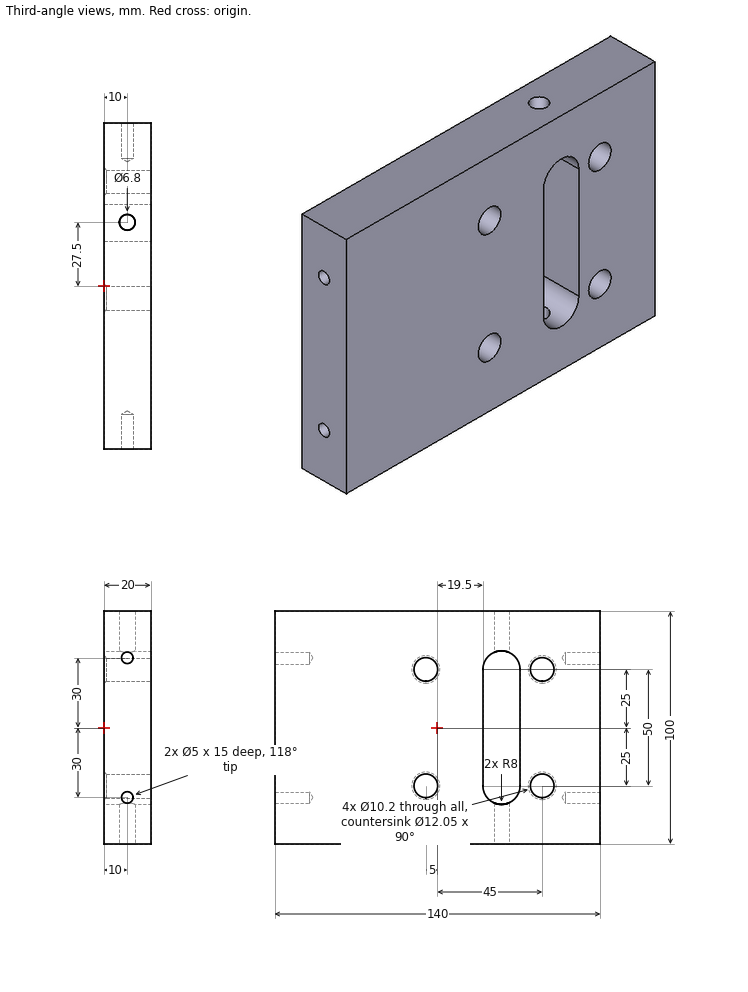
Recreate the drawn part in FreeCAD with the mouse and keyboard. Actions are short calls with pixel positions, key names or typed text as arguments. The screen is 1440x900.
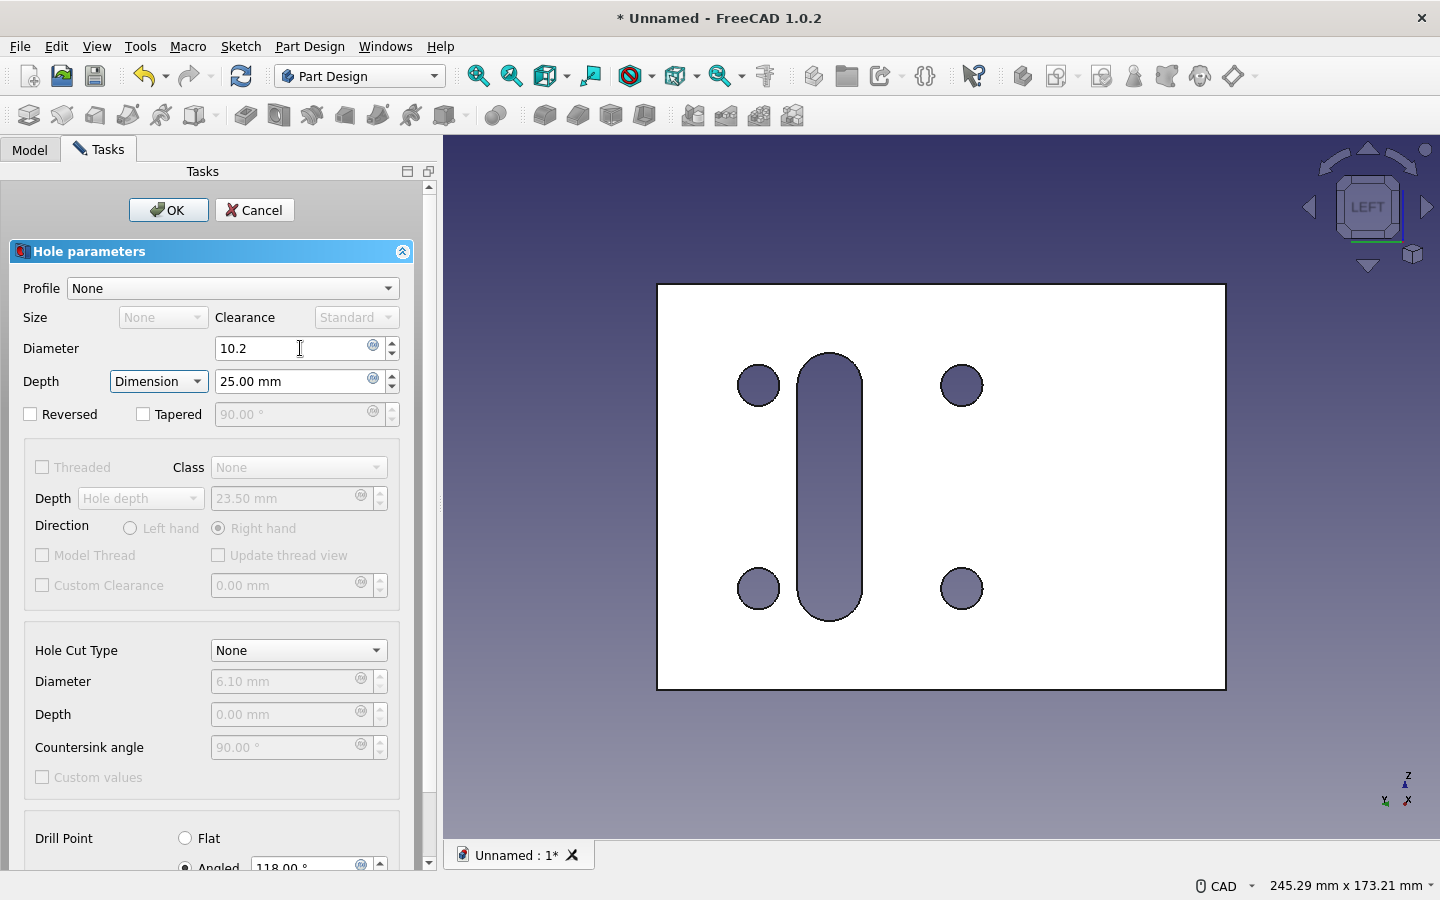
click(160, 382)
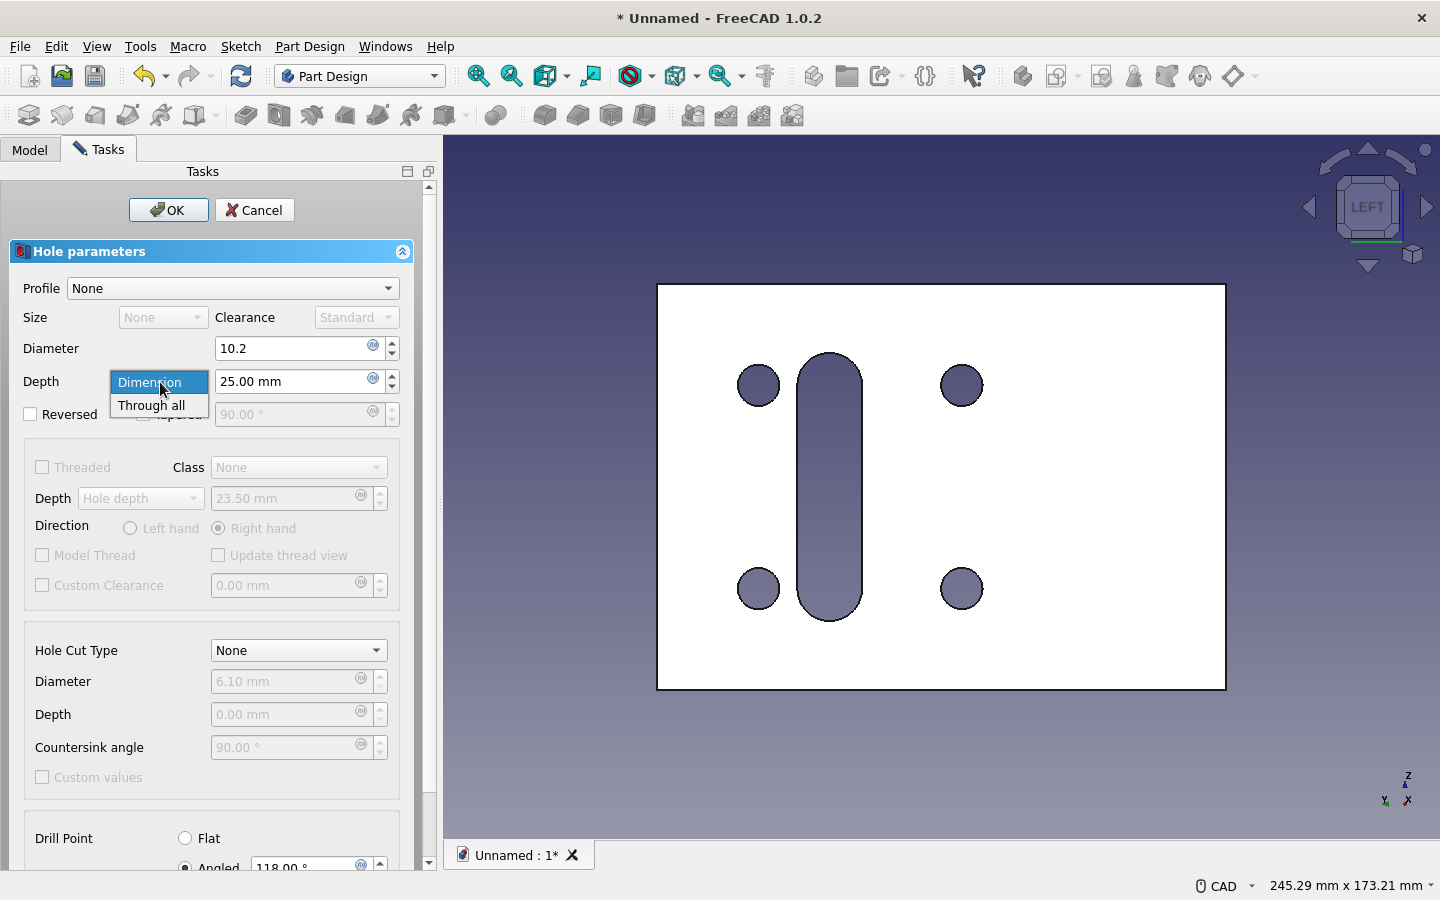
click(158, 406)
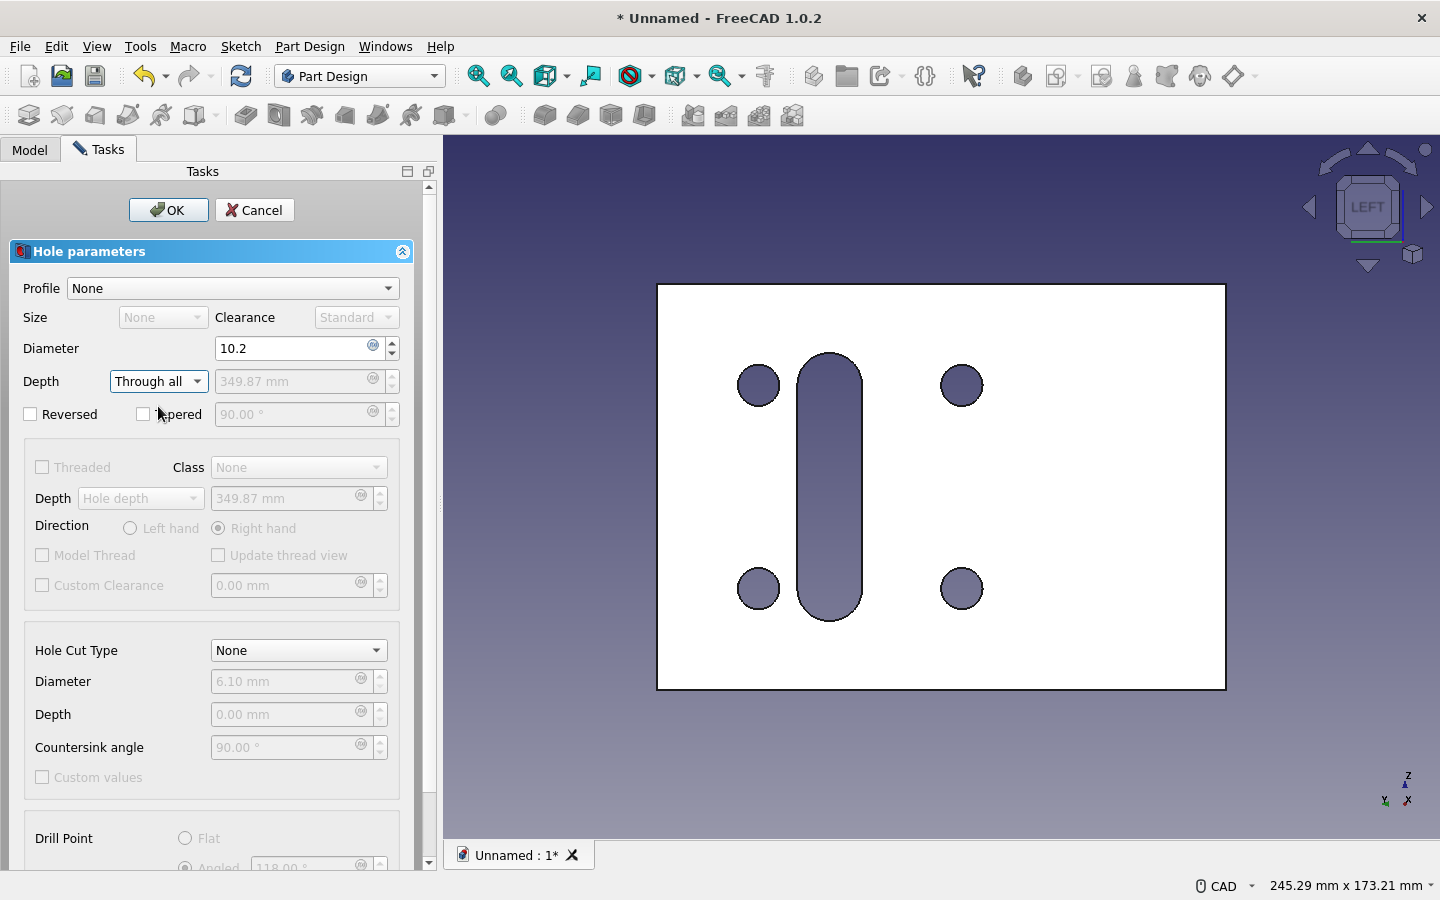
click(300, 650)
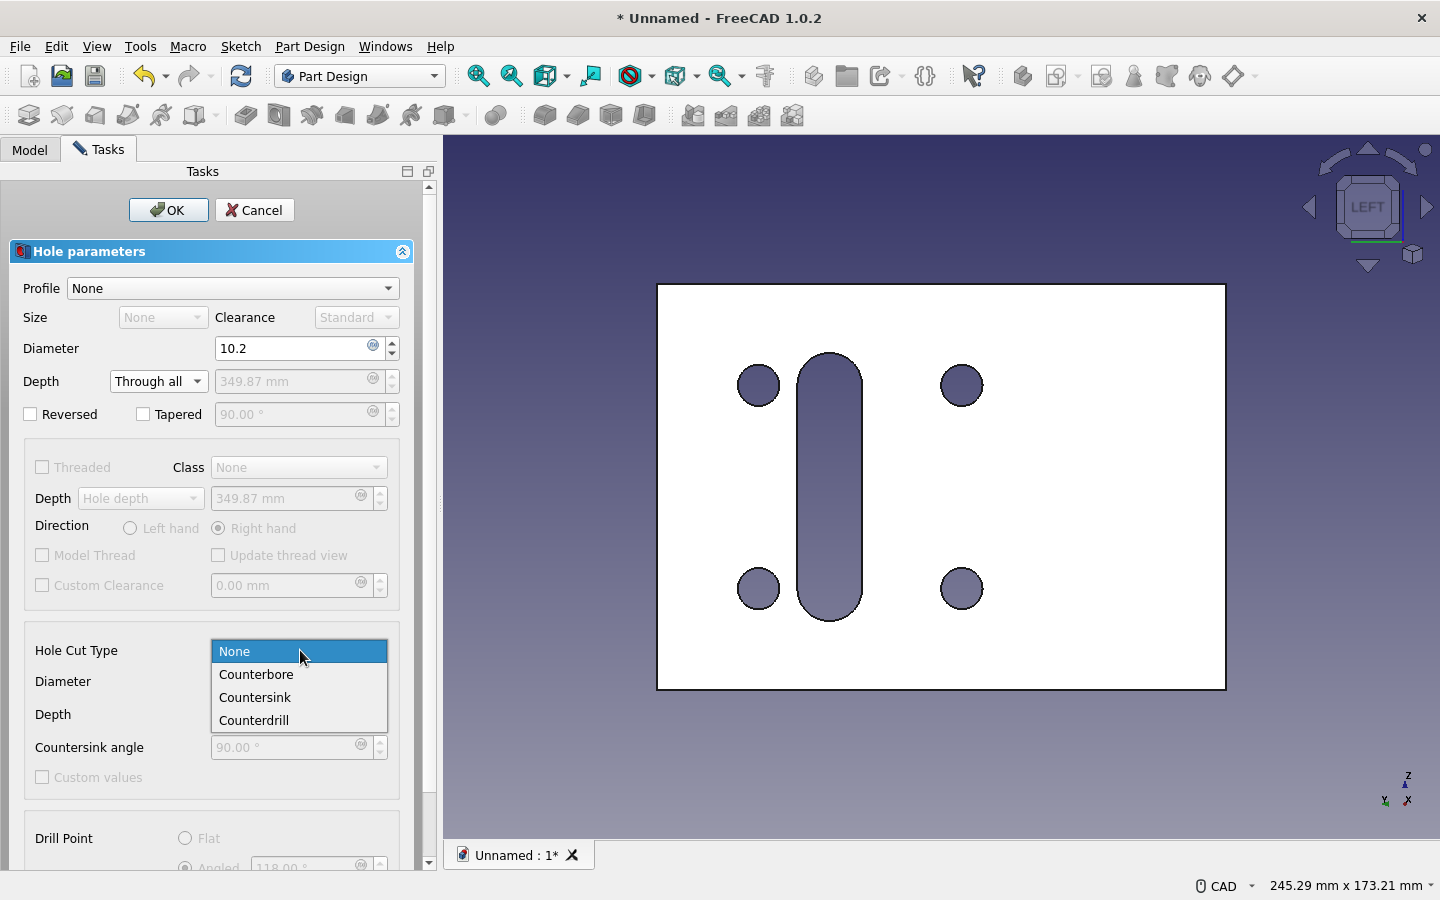
click(298, 698)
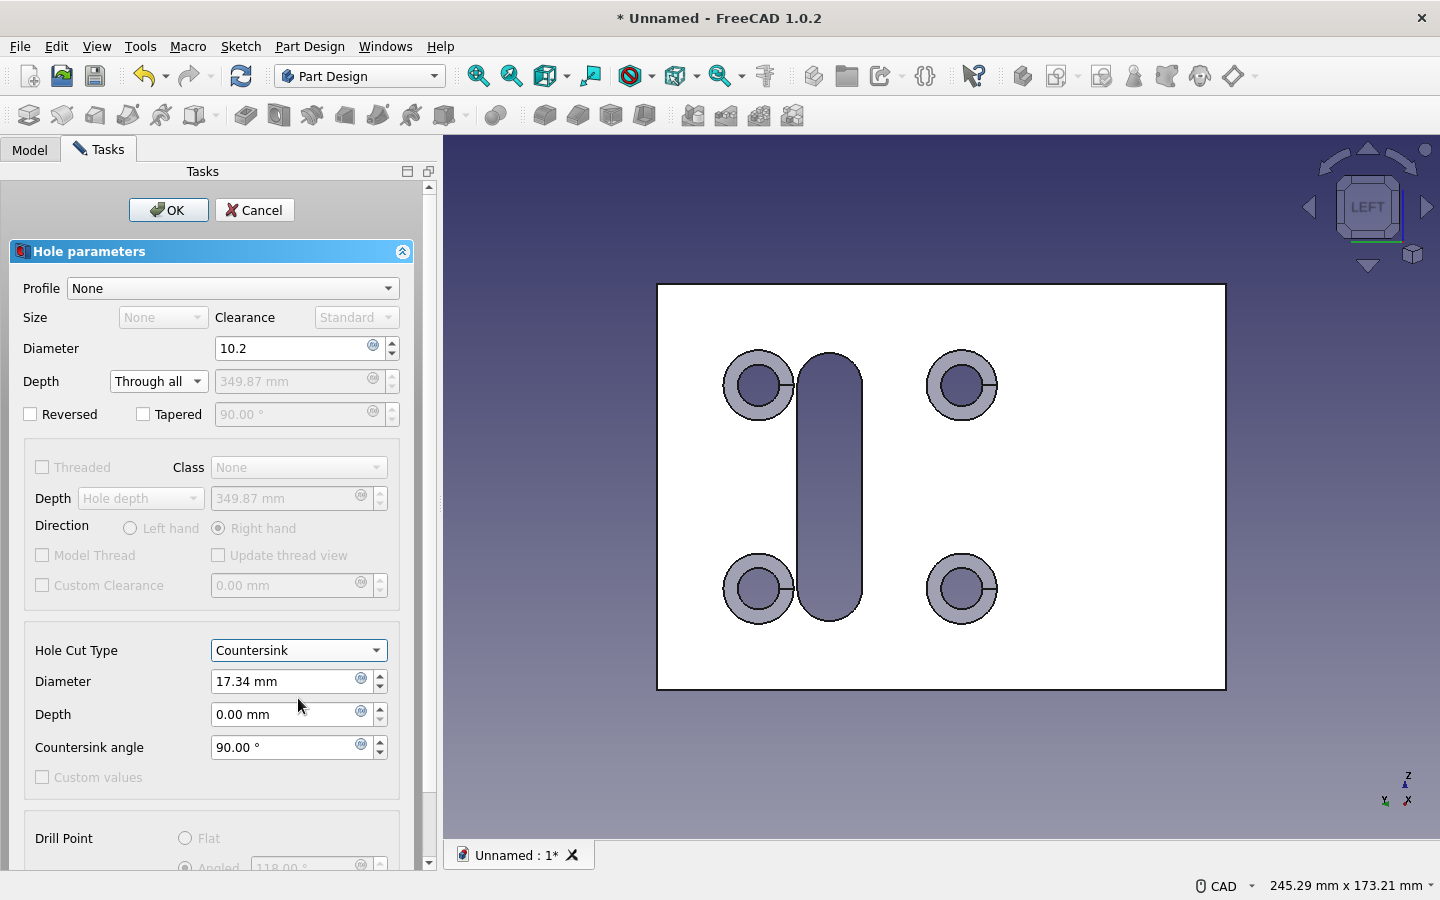
triple_click(292, 682)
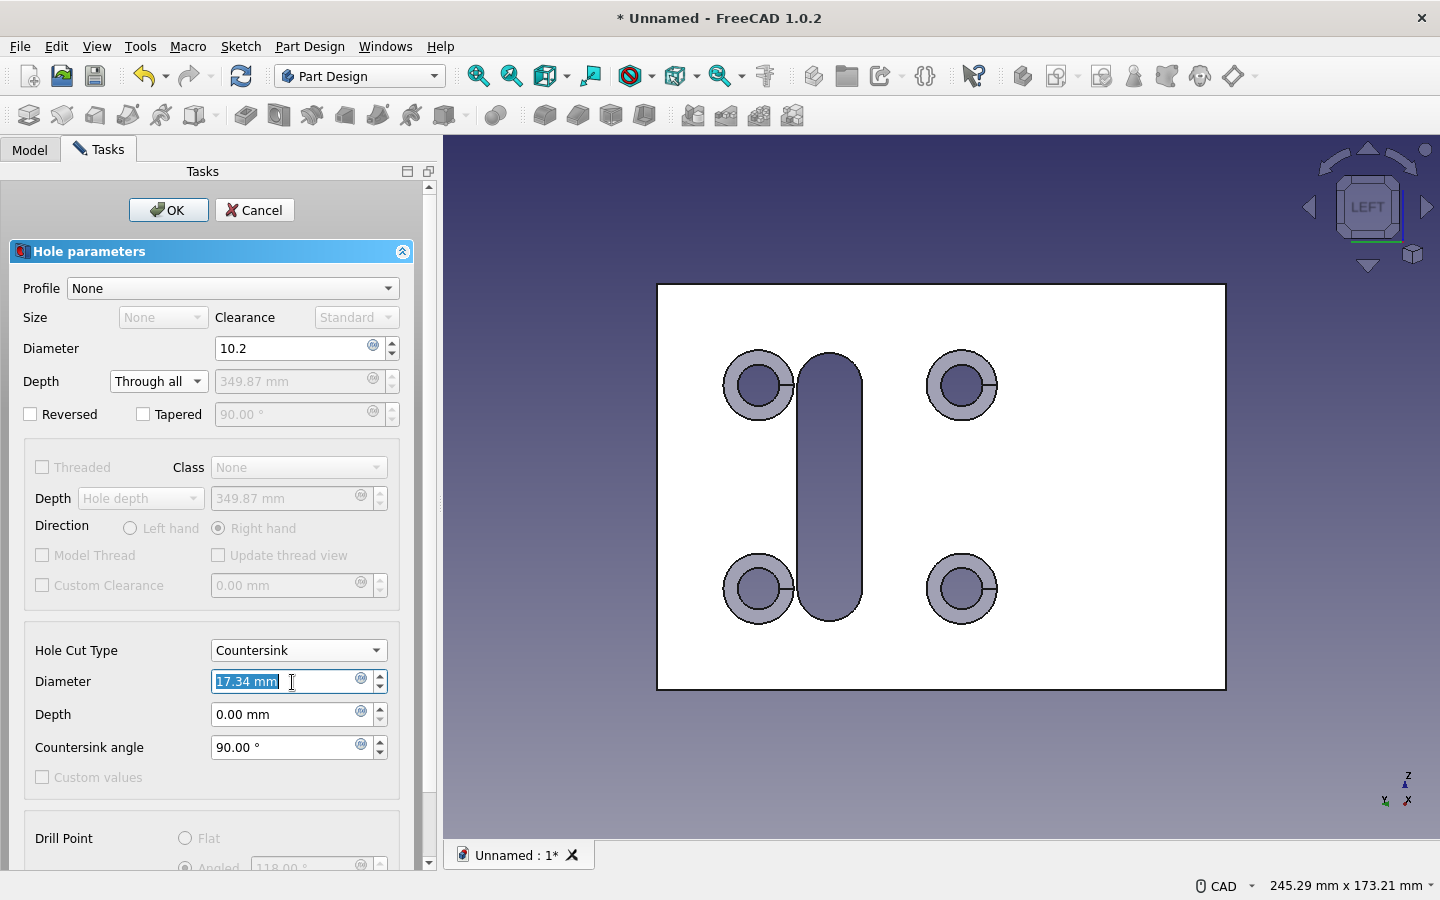
text(12.05)
key(Tab)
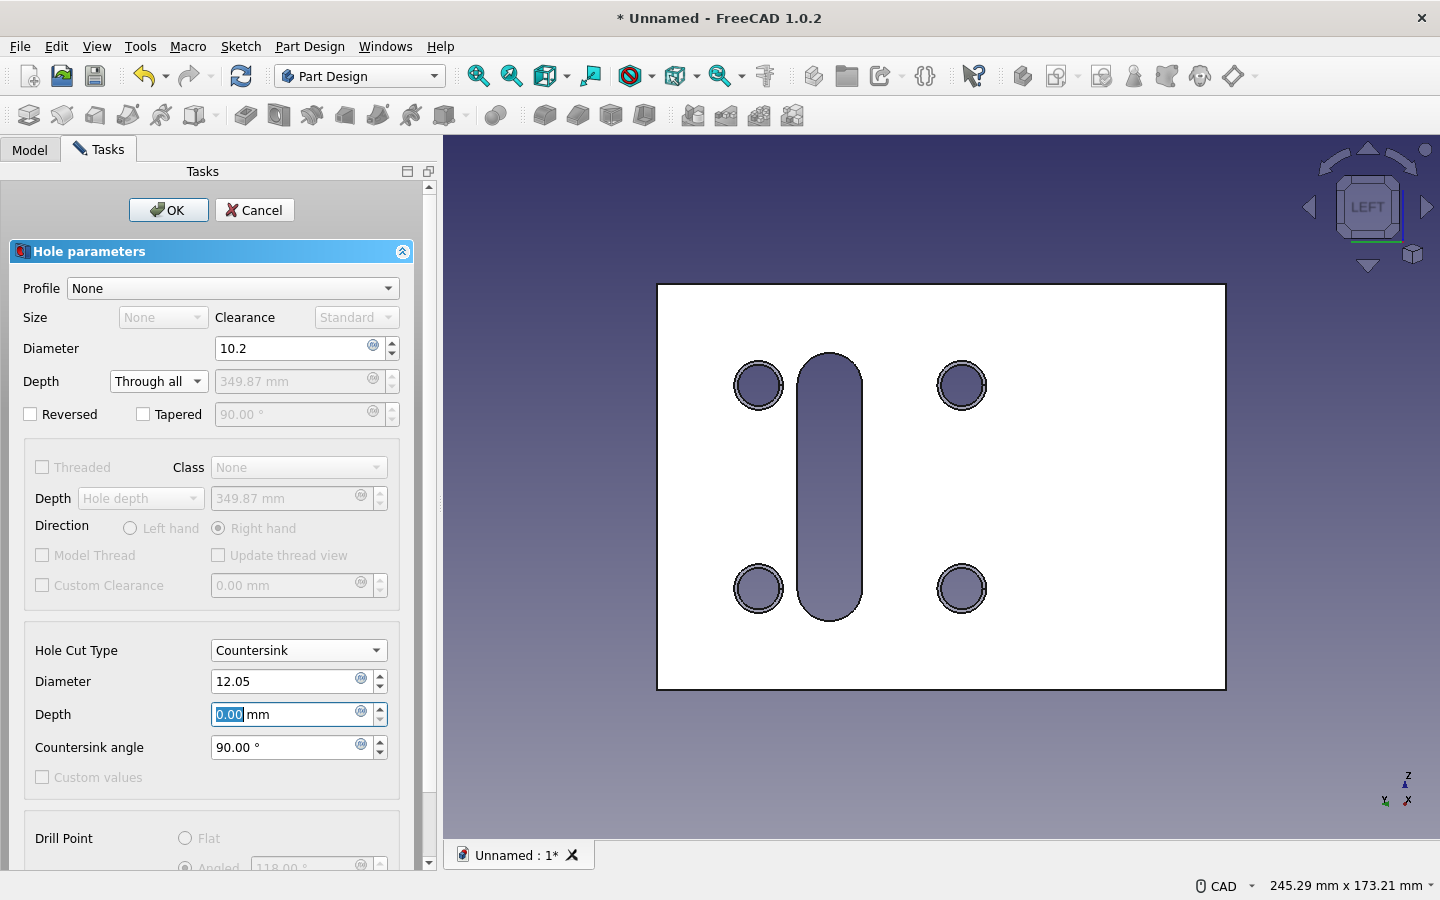
click(169, 210)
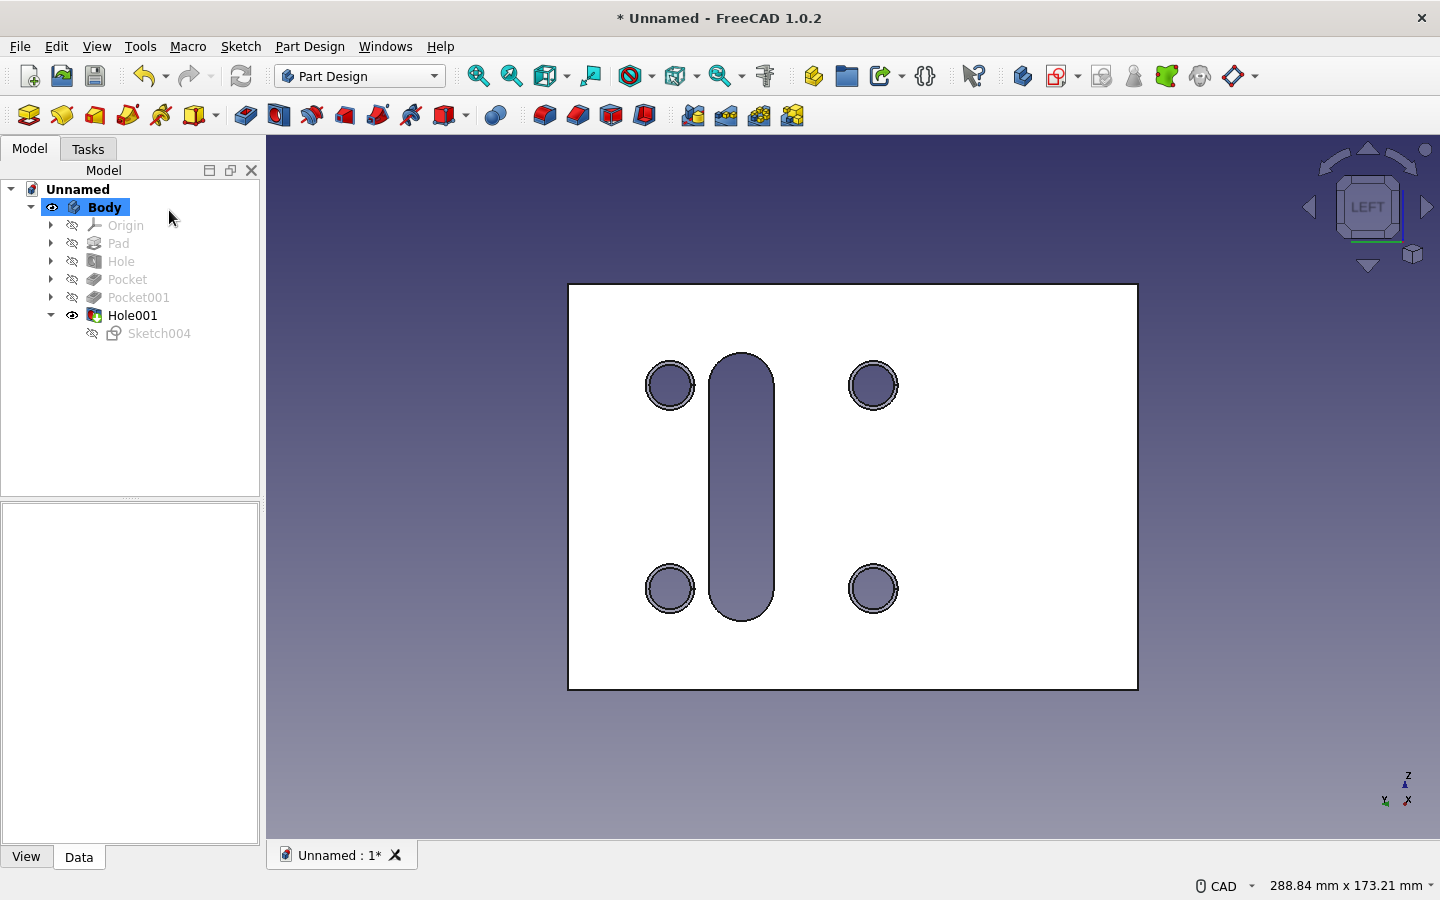
key(4)